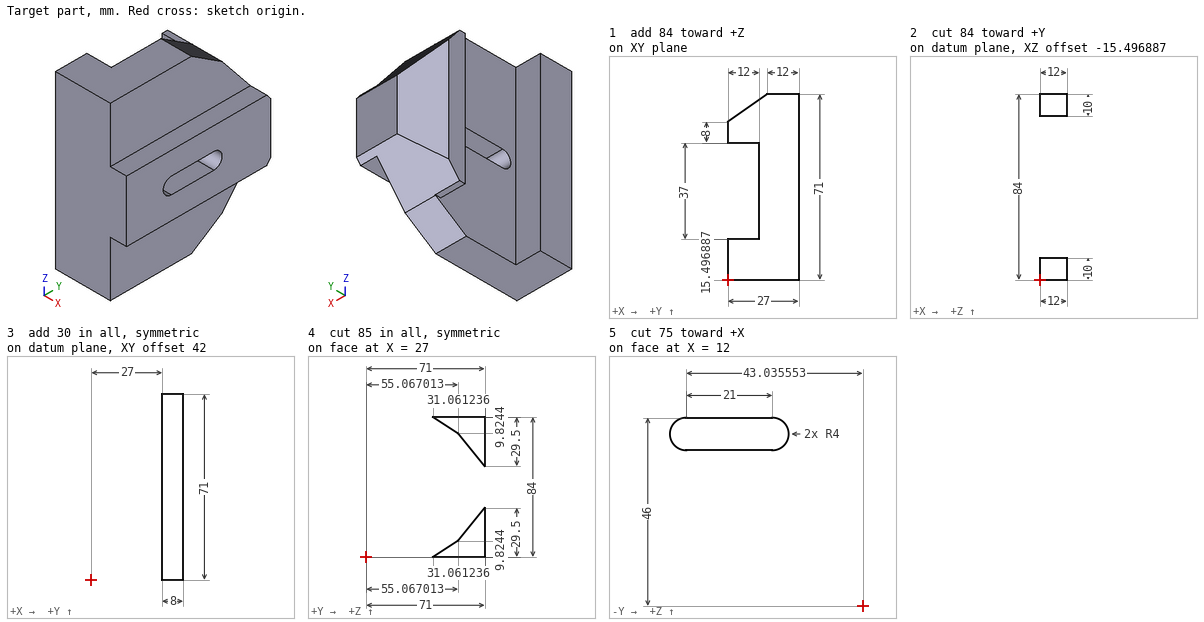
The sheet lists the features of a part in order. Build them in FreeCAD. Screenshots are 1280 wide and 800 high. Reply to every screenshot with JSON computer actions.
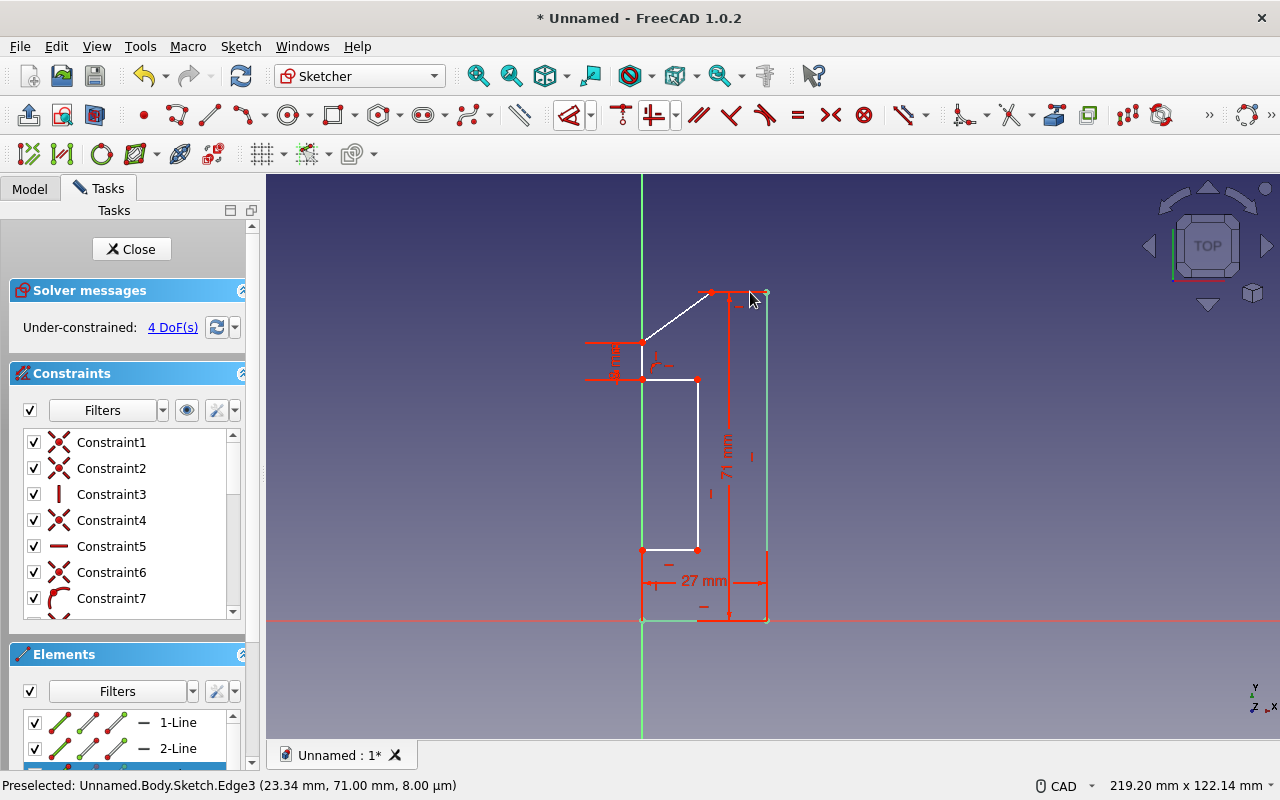
{"action": "key", "text": "l"}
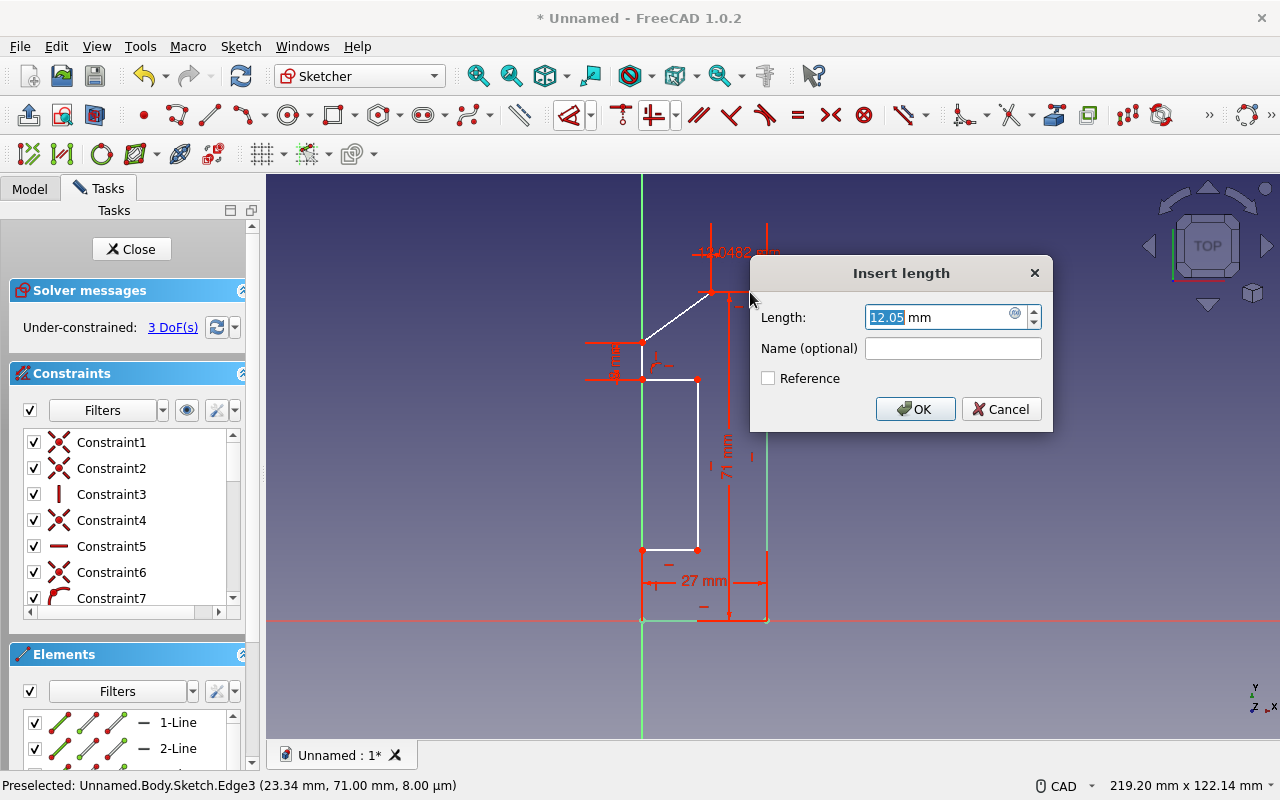
{"action": "type", "text": "12"}
{"action": "key", "text": "Return"}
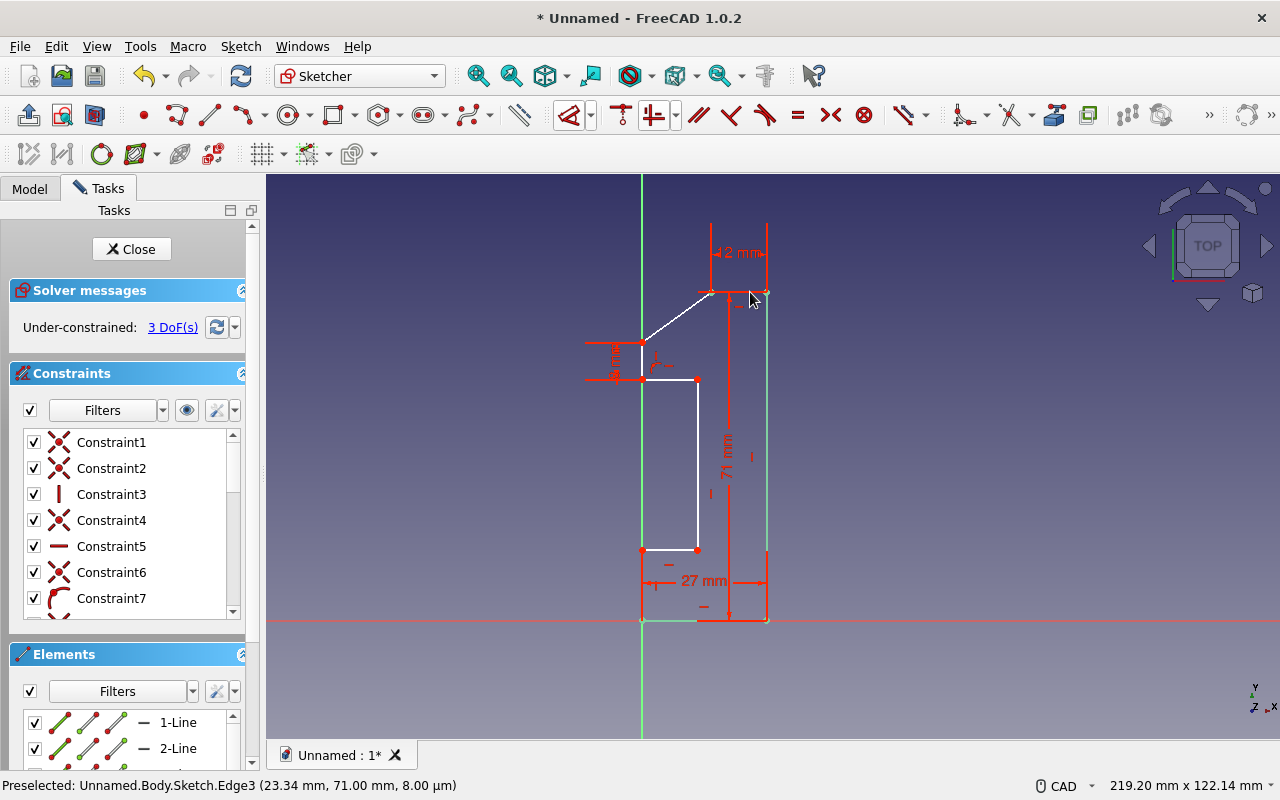
{"action": "left_click", "coordinate": [659, 380]}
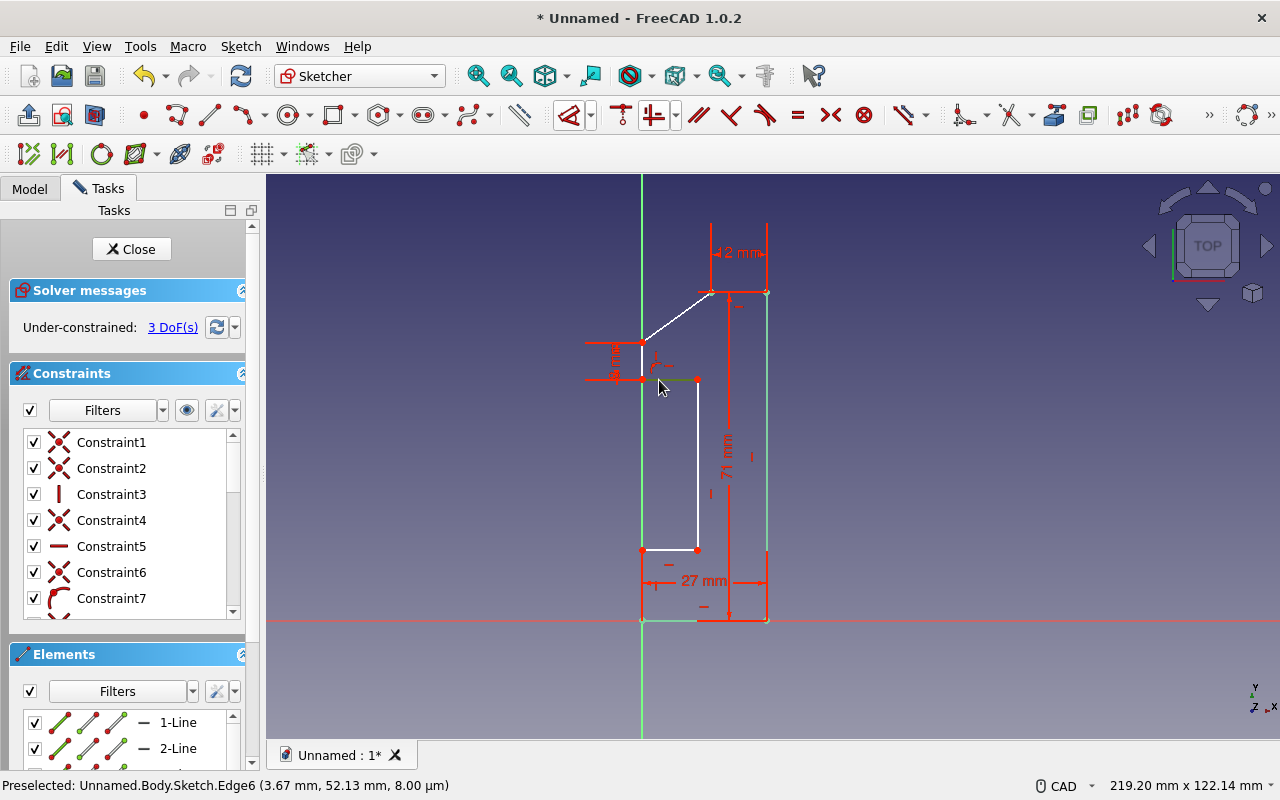
{"action": "key", "text": "l"}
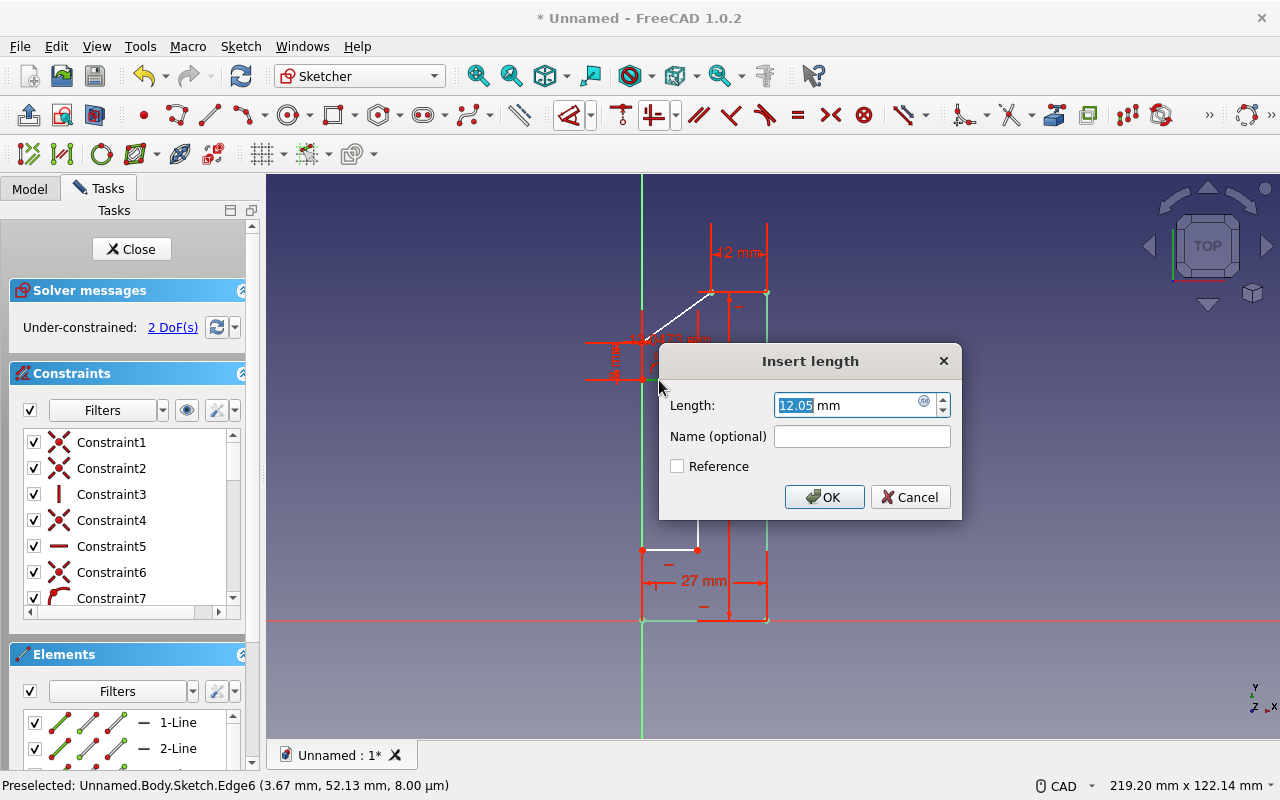
{"action": "type", "text": "12"}
{"action": "key", "text": "Return"}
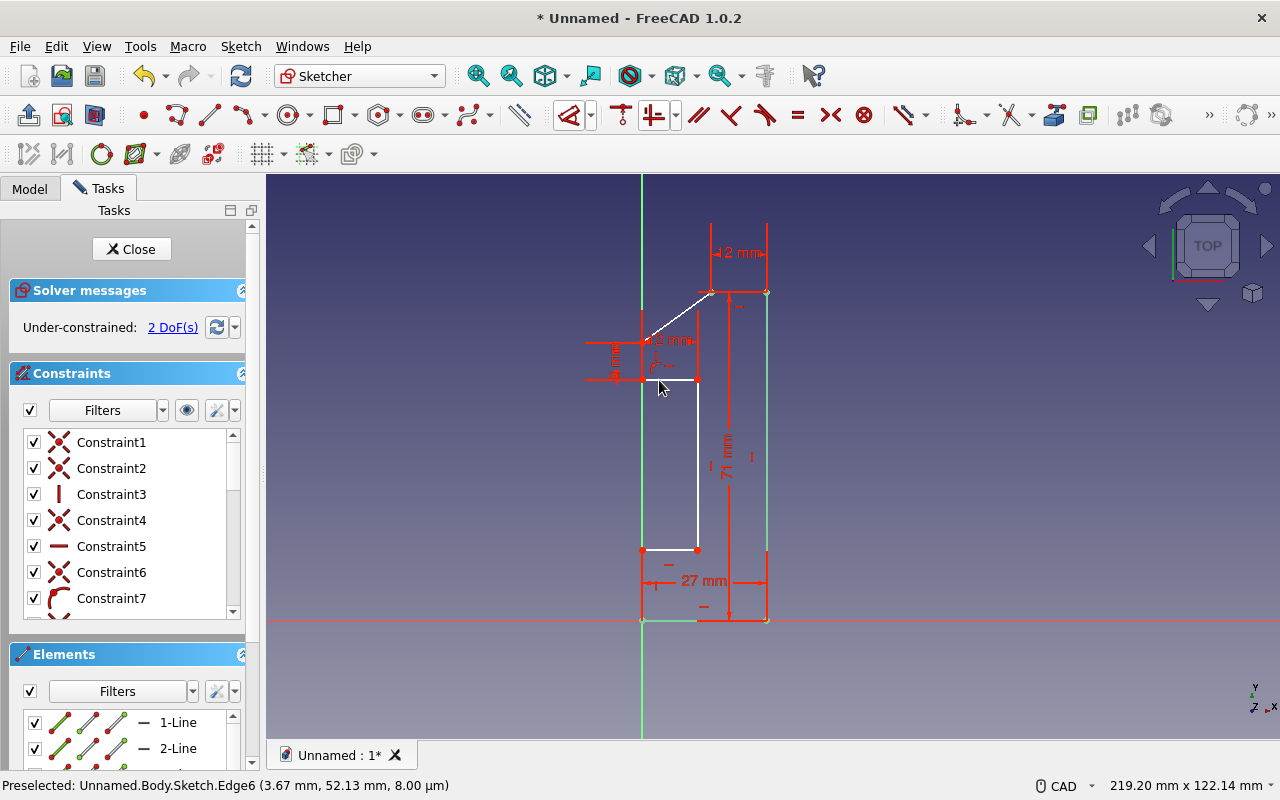
{"action": "left_click", "coordinate": [698, 431]}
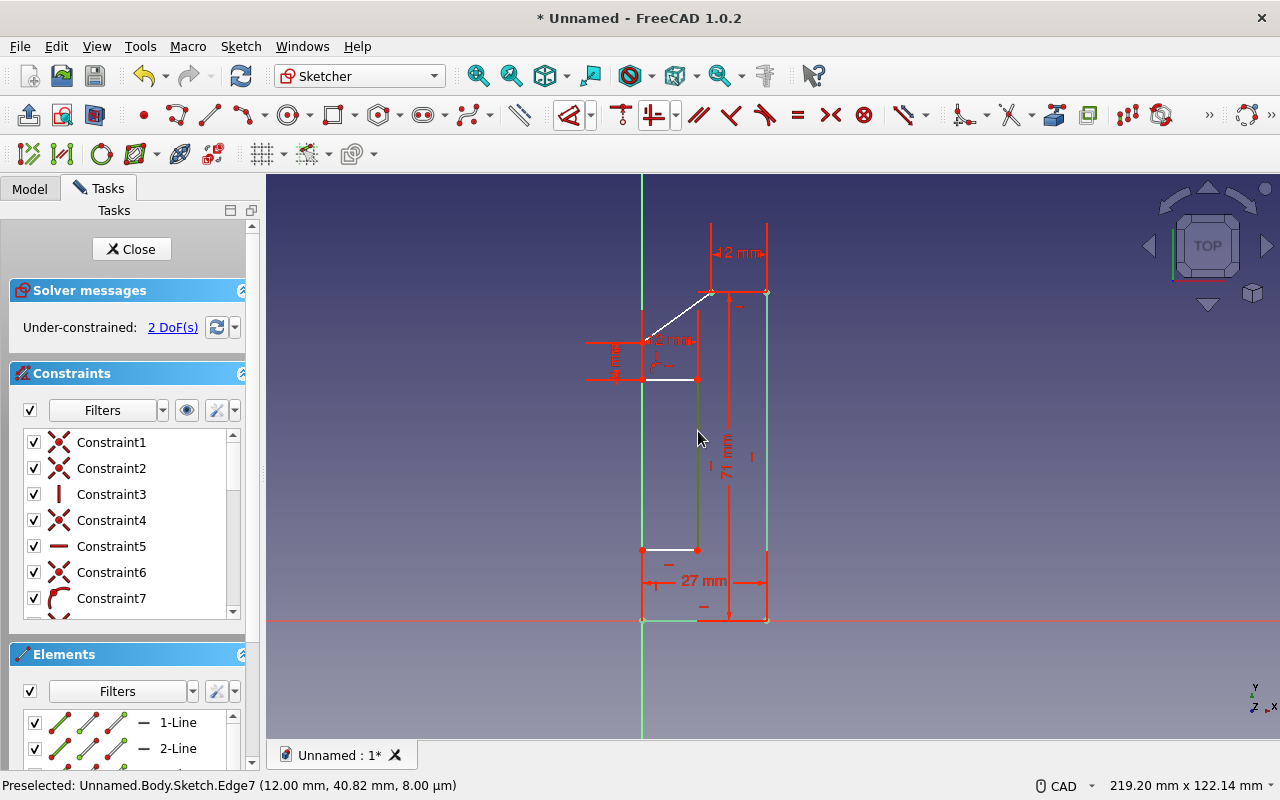
{"action": "left_click", "coordinate": [590, 116]}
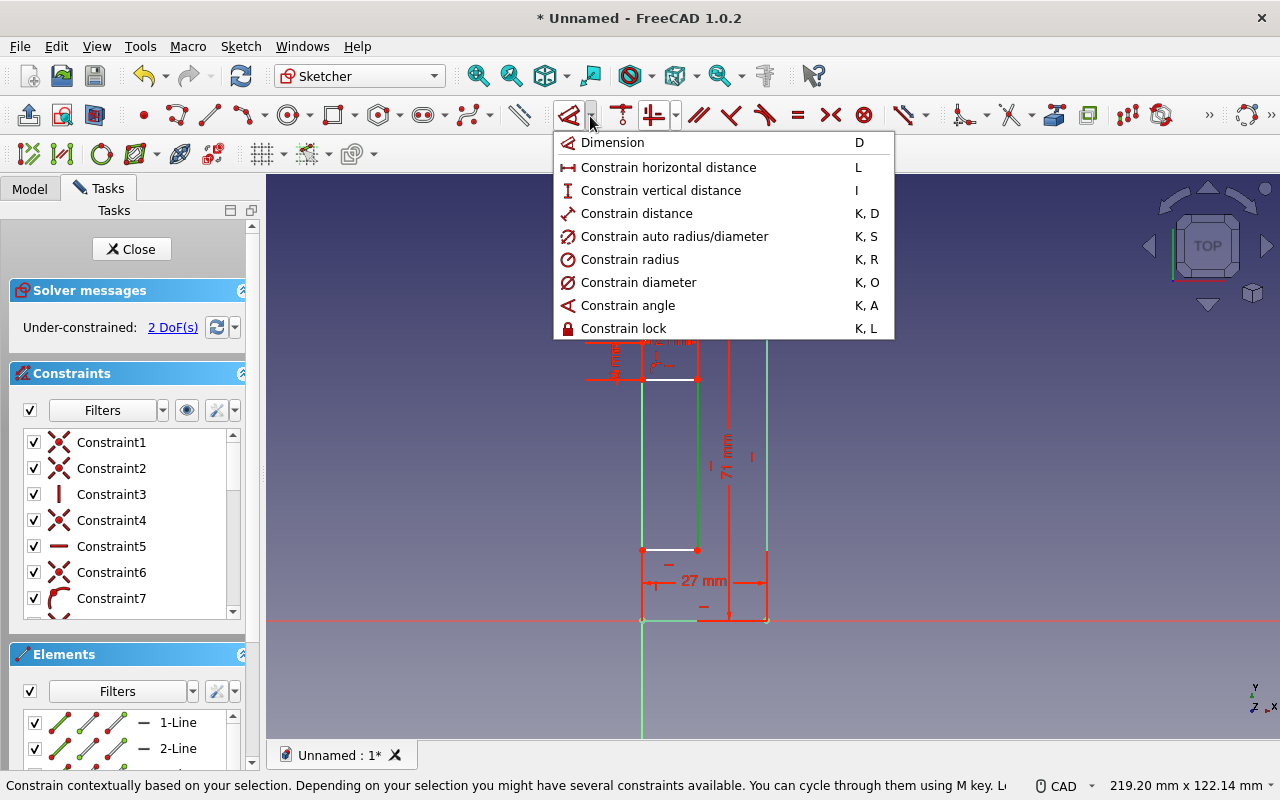
{"action": "left_click", "coordinate": [724, 190]}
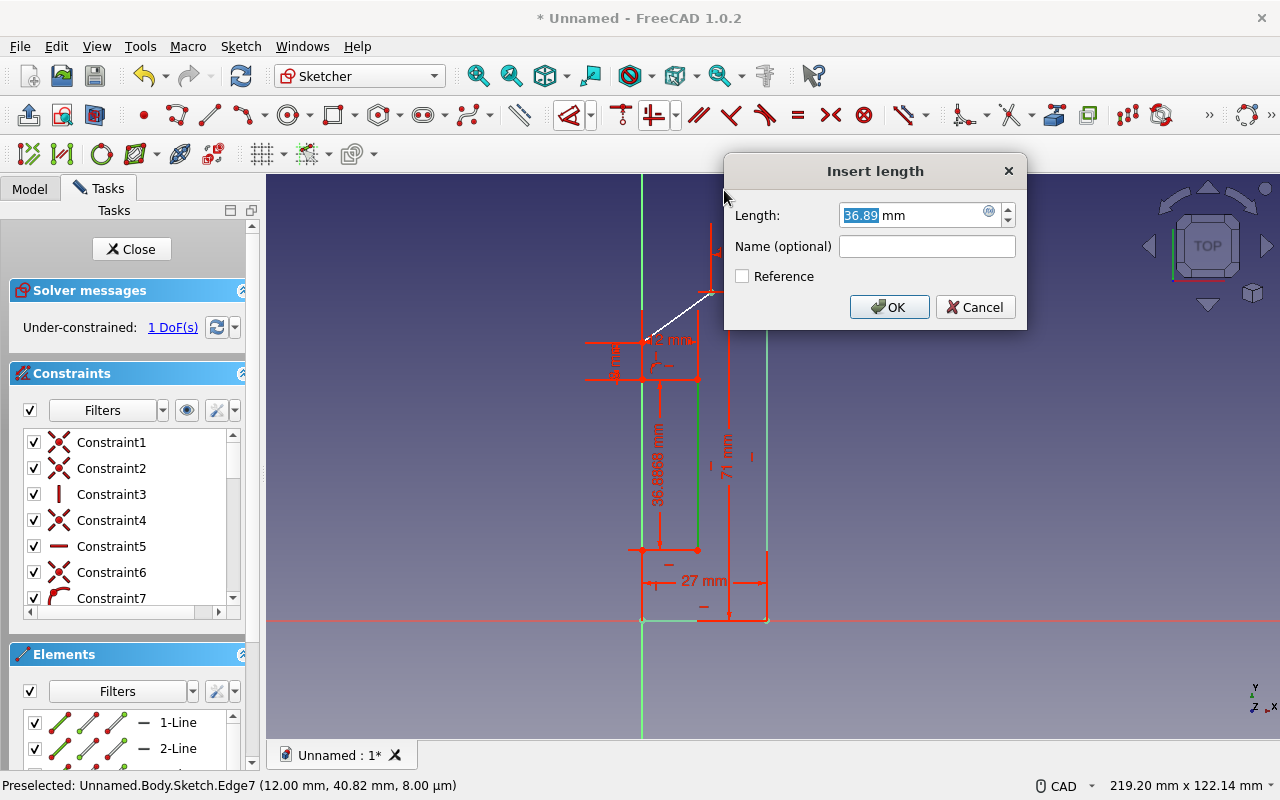
{"action": "type", "text": "37"}
{"action": "key", "text": "Return"}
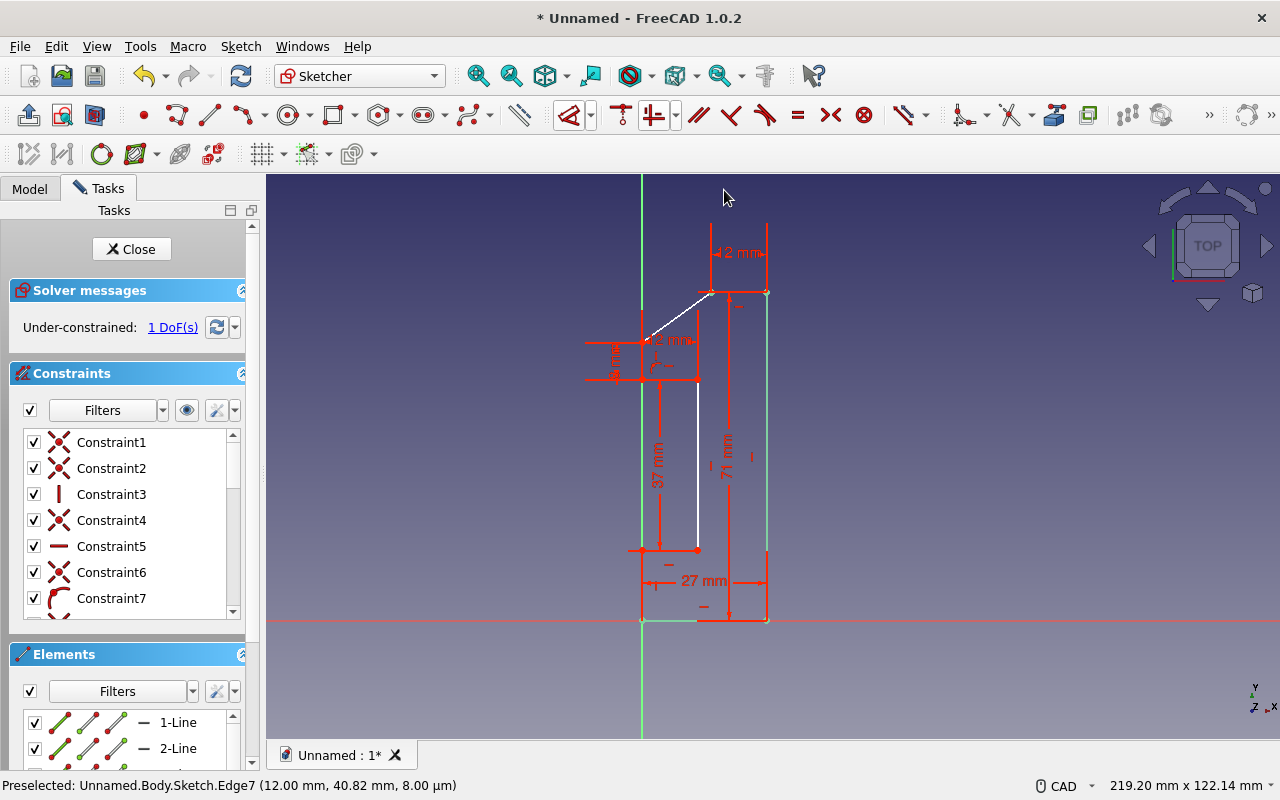
{"action": "left_click", "coordinate": [642, 572]}